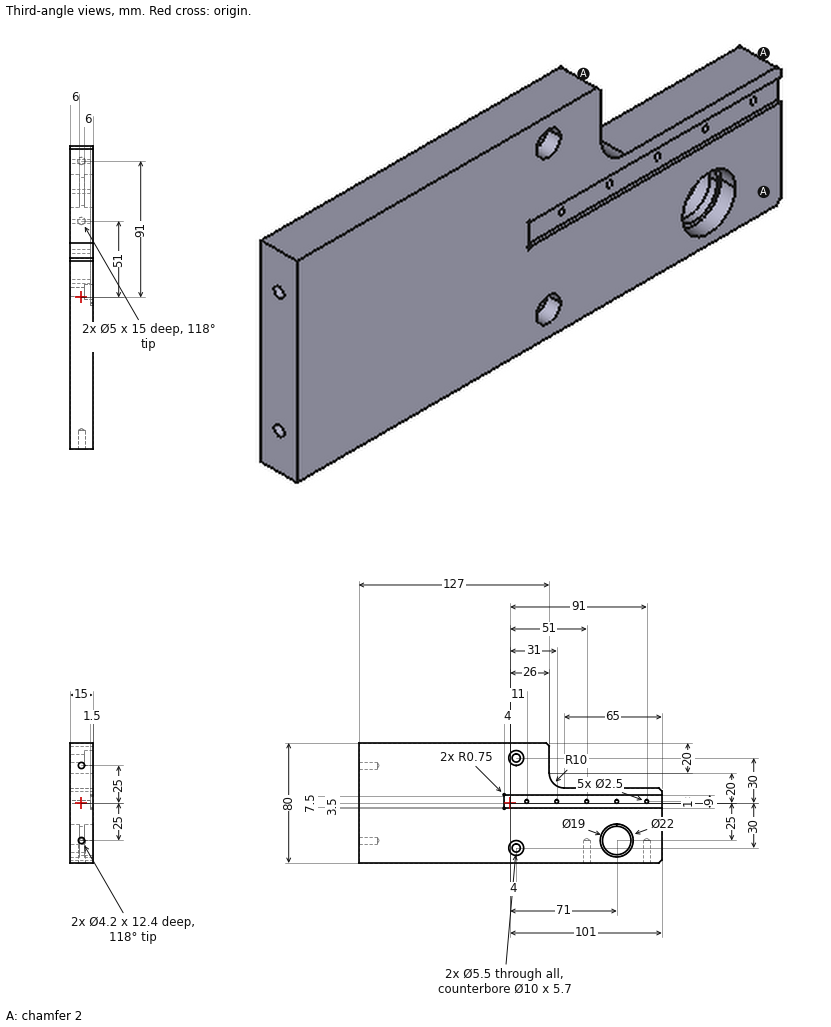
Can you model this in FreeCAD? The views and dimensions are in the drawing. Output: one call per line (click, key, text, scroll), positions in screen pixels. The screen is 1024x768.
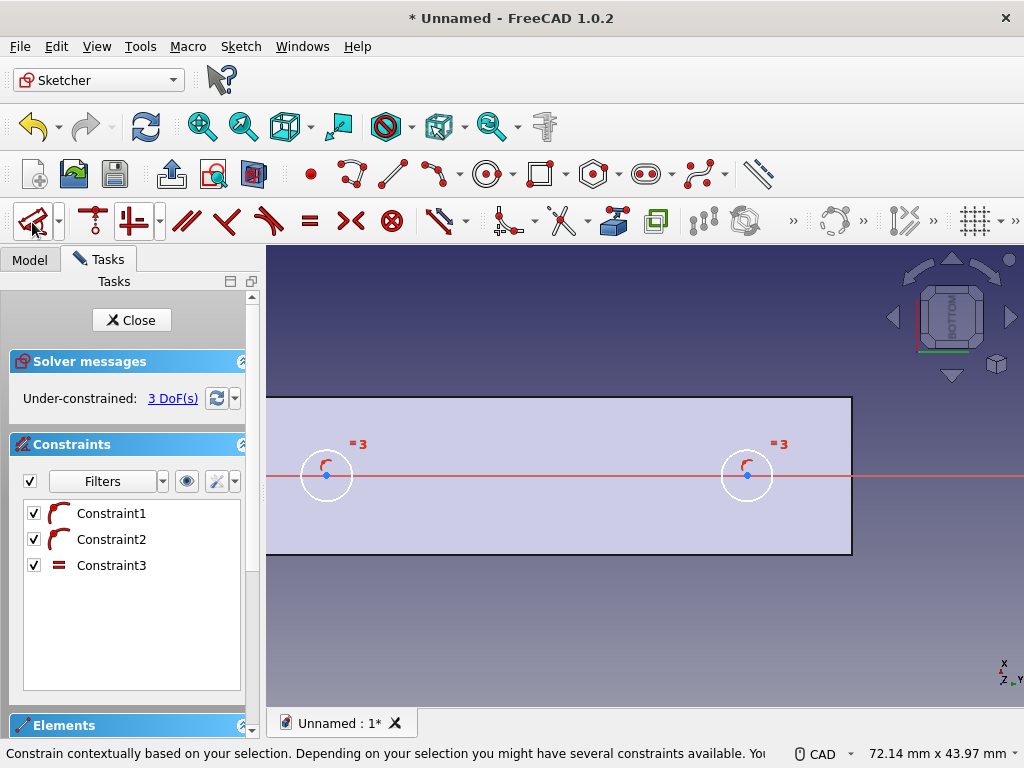
click(345, 458)
click(368, 436)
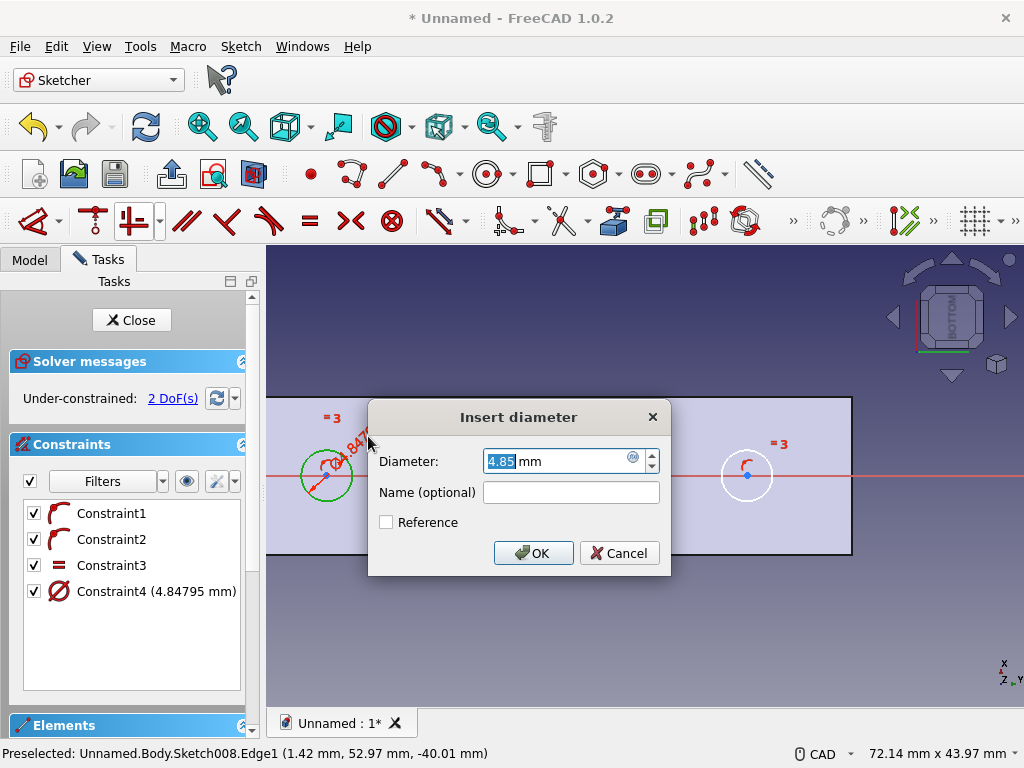
text(5)
key(Return)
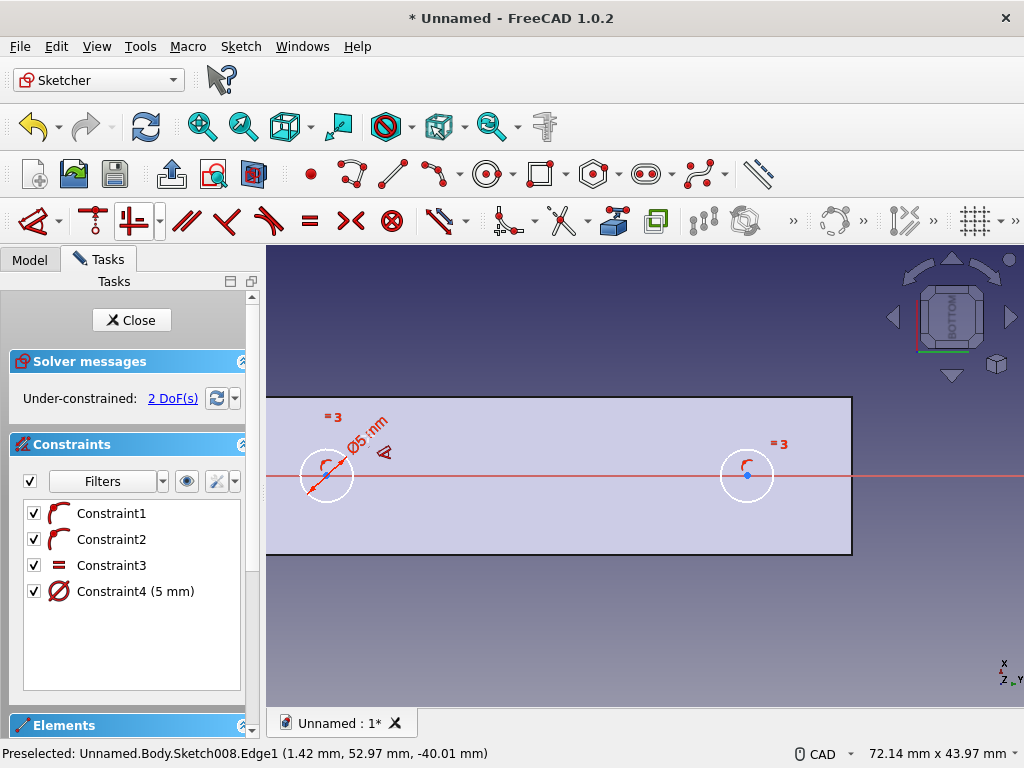
click(327, 476)
click(303, 510)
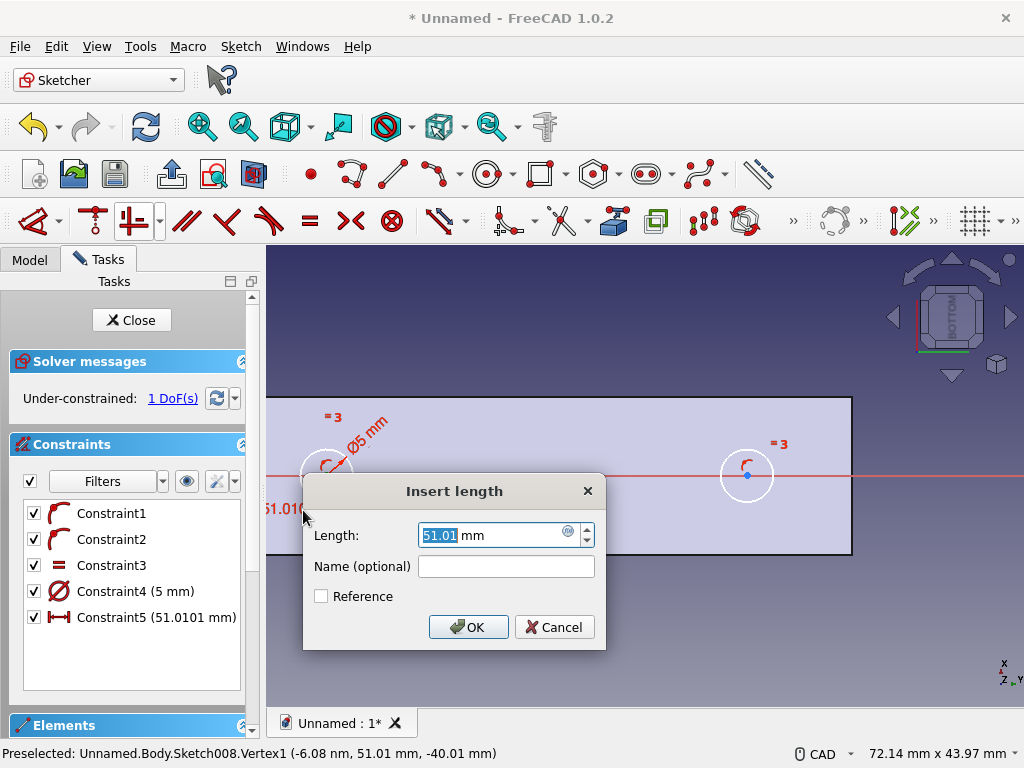
text(51)
key(Return)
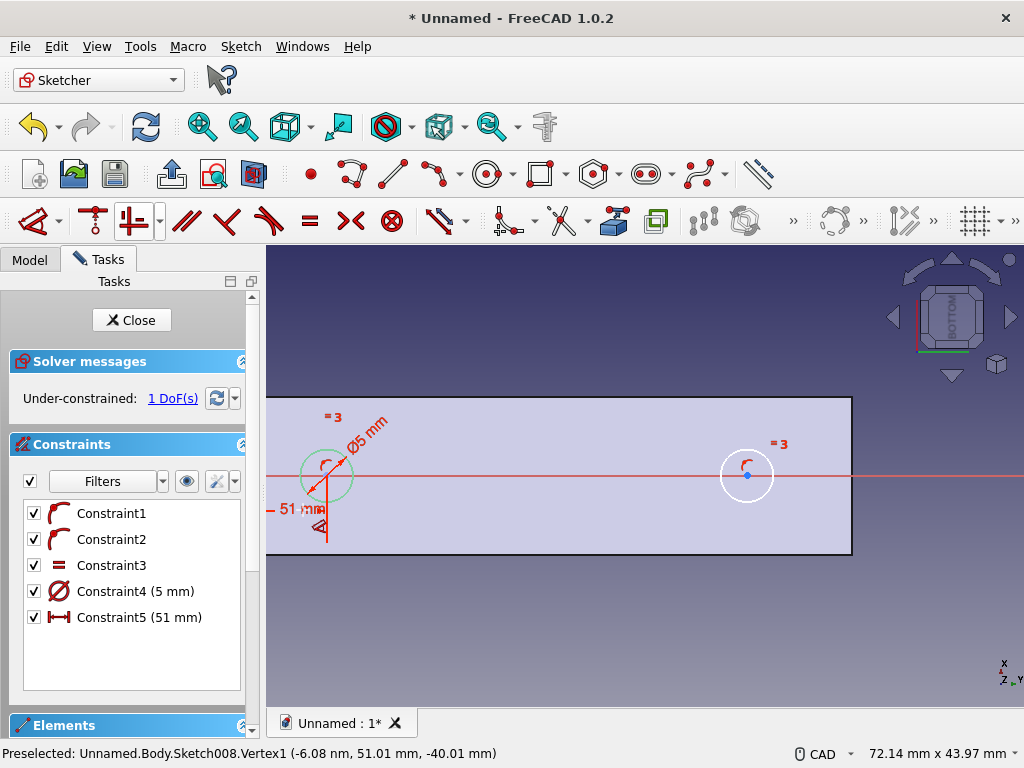
click(747, 476)
click(520, 510)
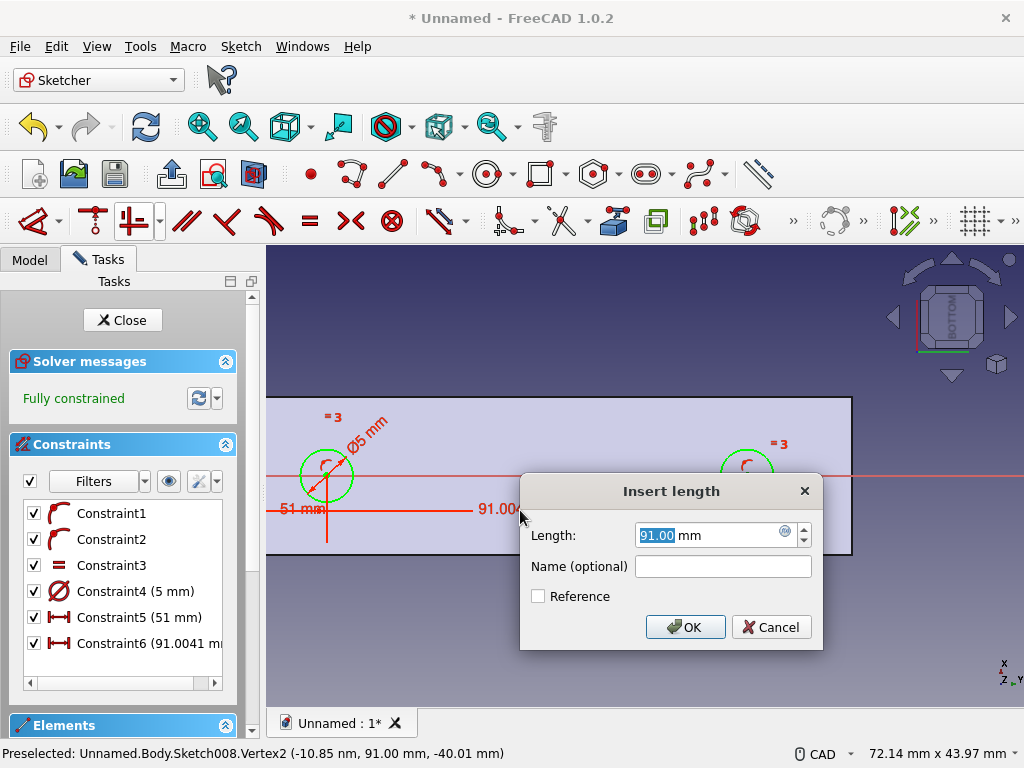
text(91)
key(Return)
key(Escape)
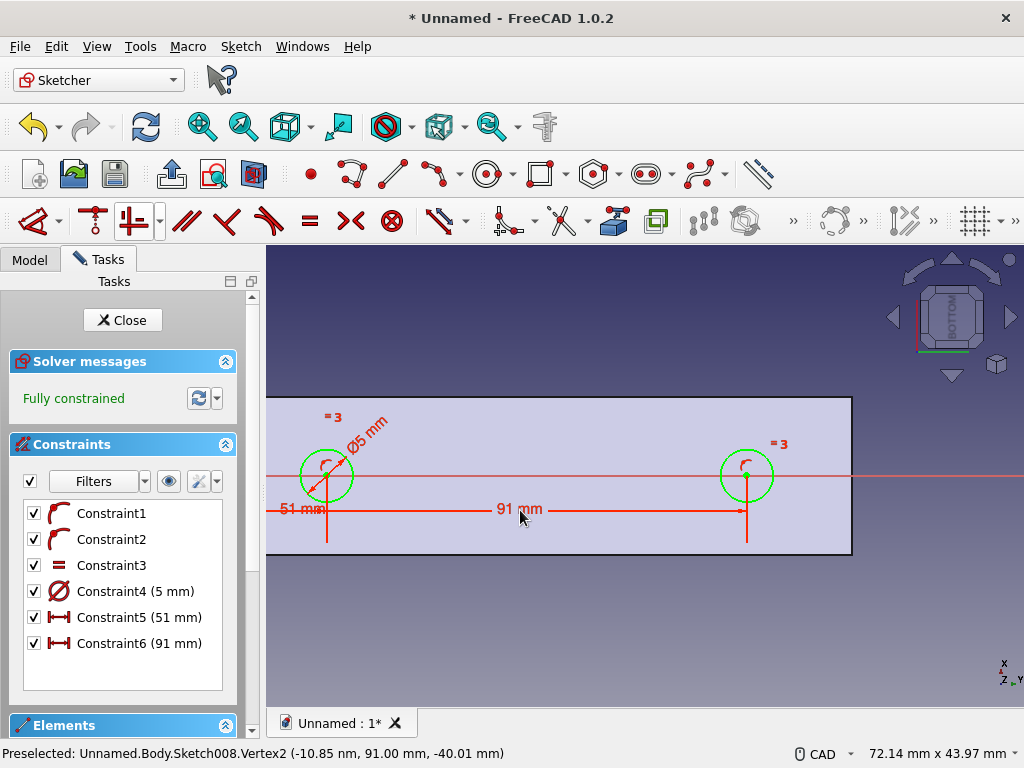
click(123, 320)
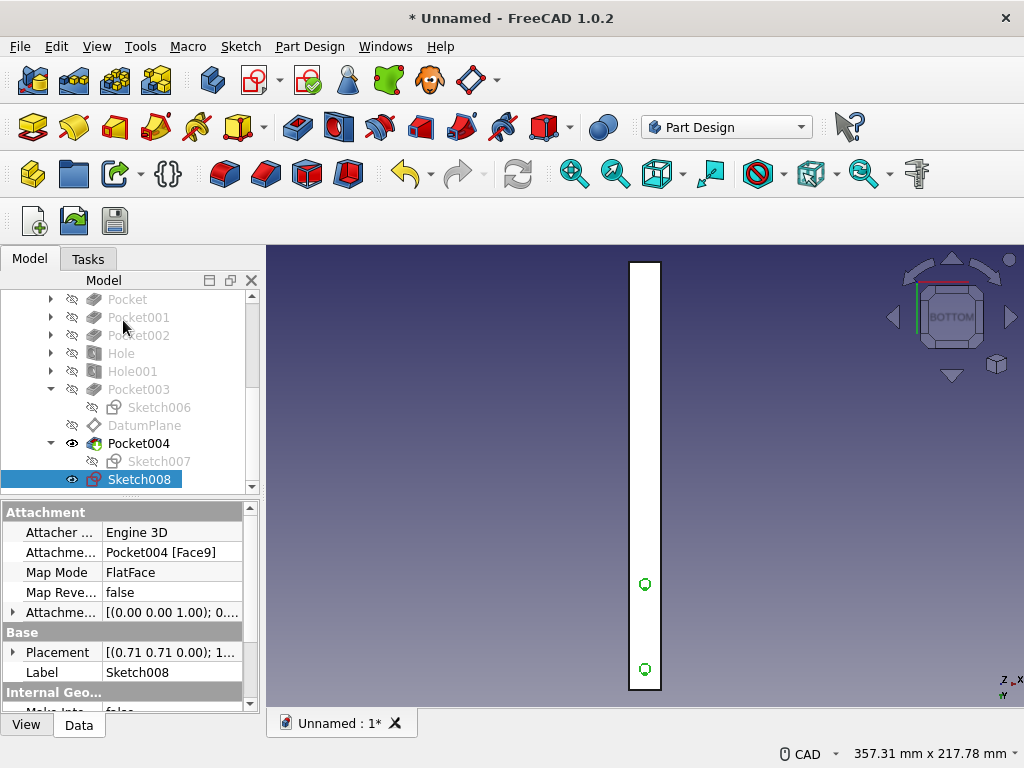
click(339, 128)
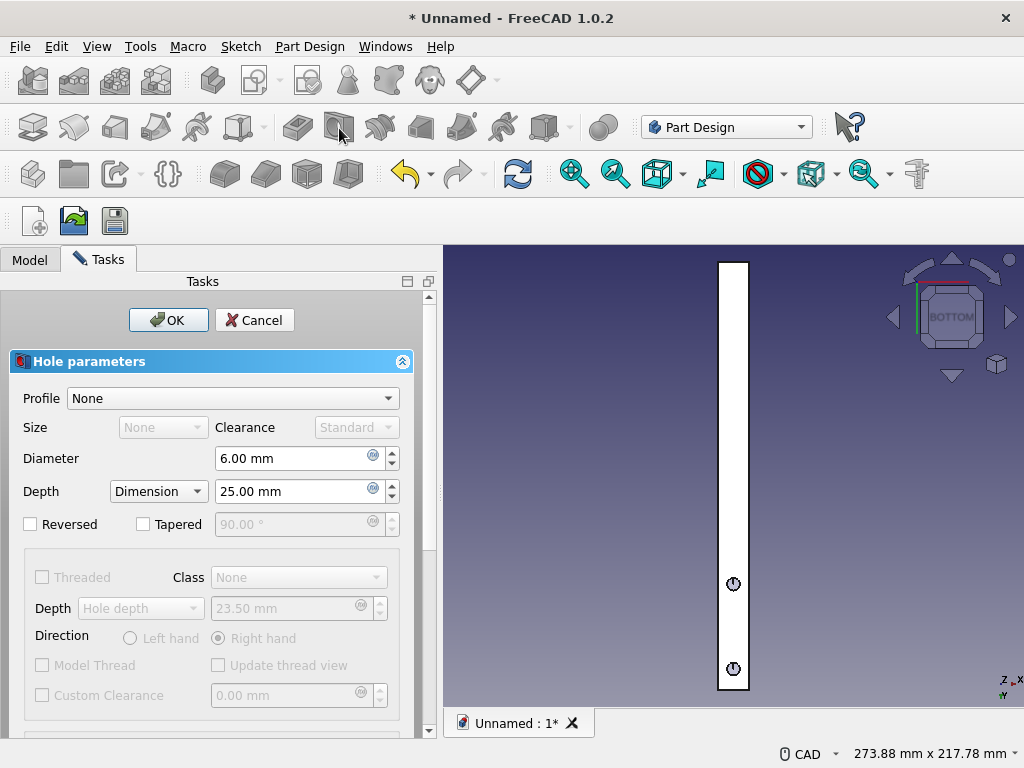
triple_click(300, 458)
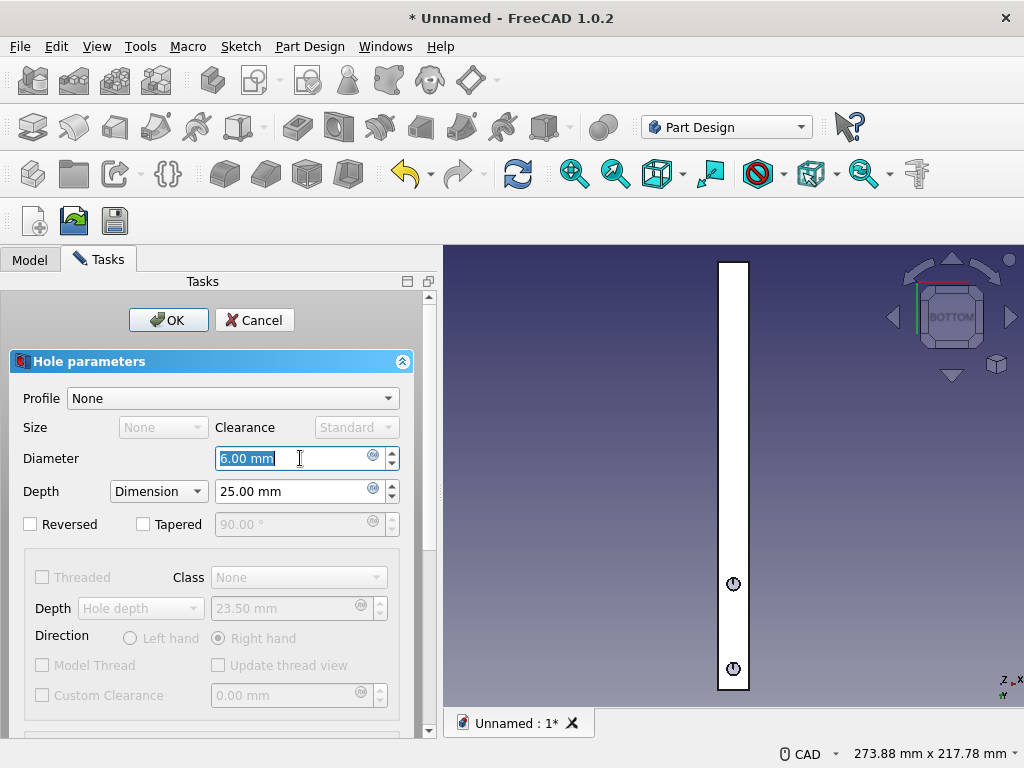
text(5)
key(Tab)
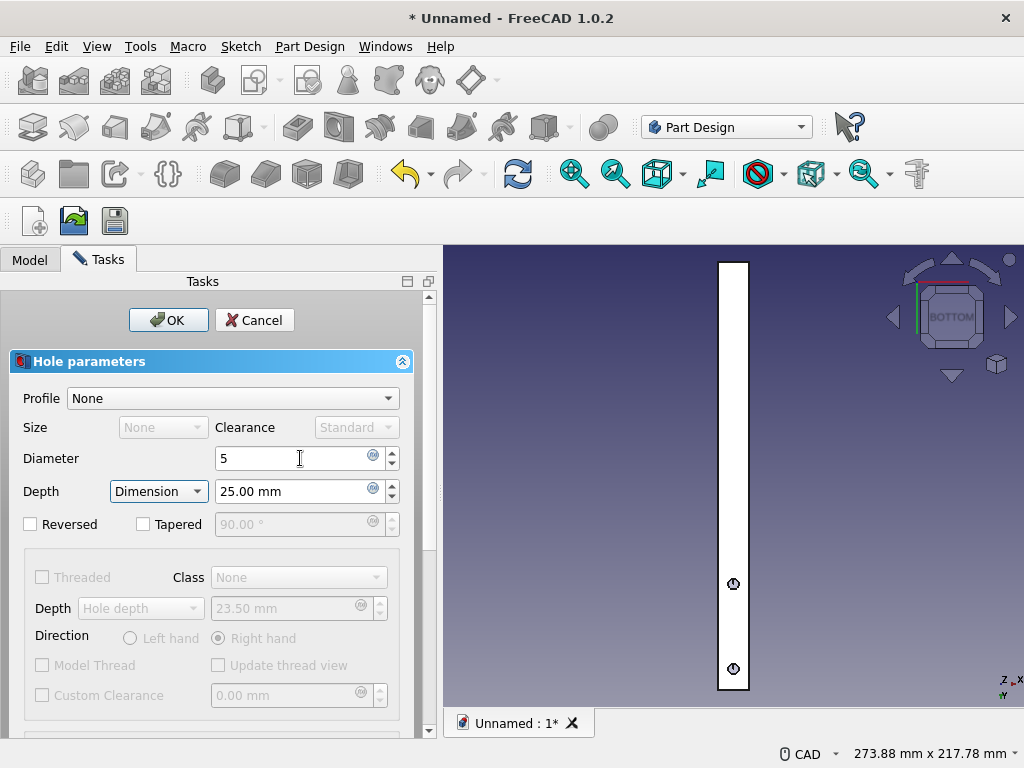
triple_click(300, 492)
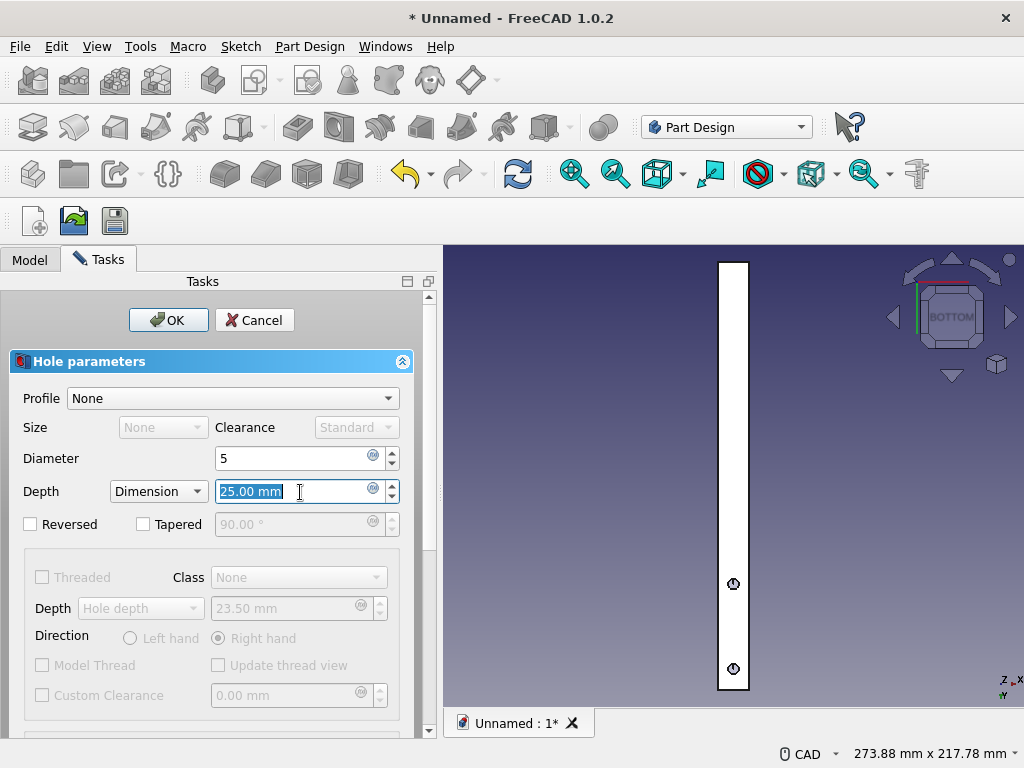
text(15)
key(Tab)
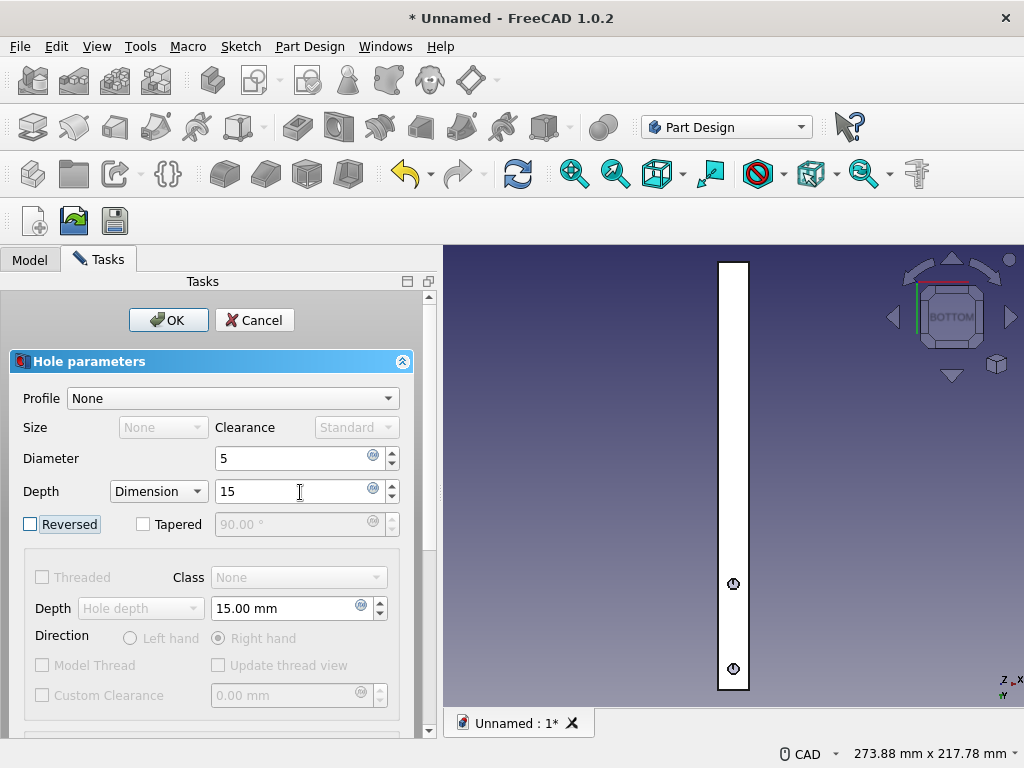
click(169, 320)